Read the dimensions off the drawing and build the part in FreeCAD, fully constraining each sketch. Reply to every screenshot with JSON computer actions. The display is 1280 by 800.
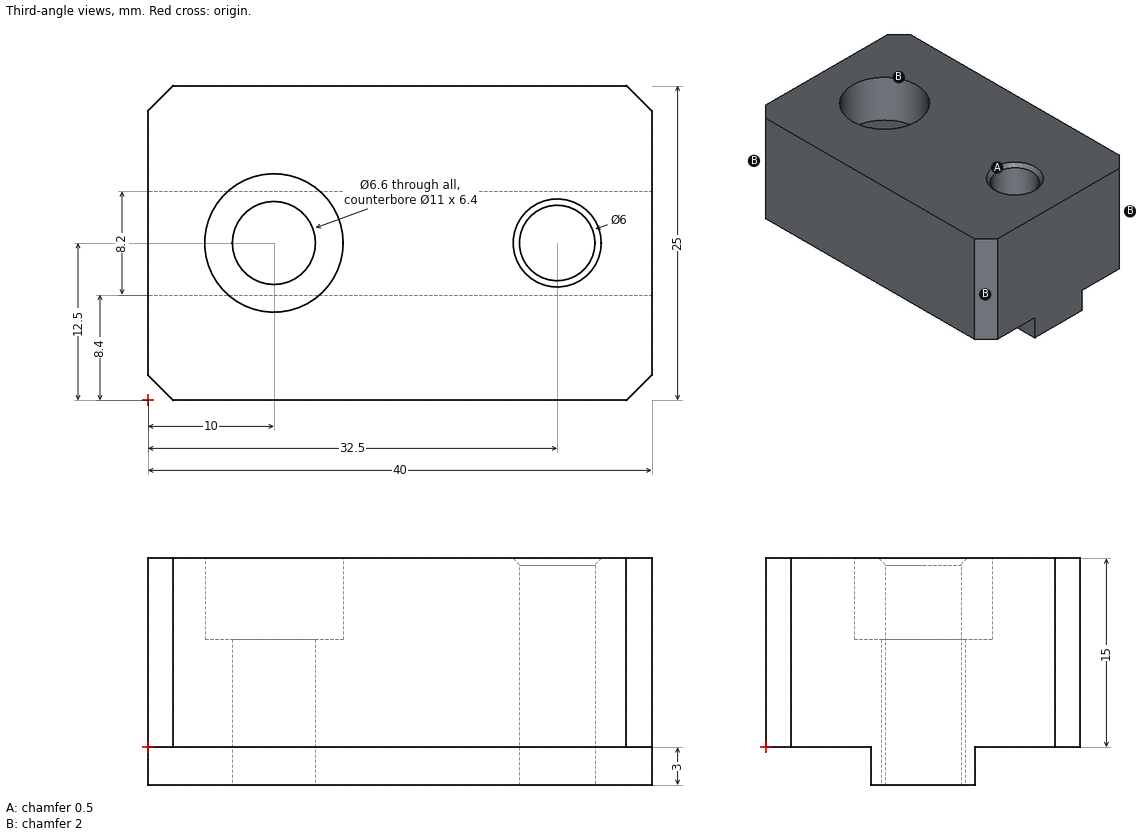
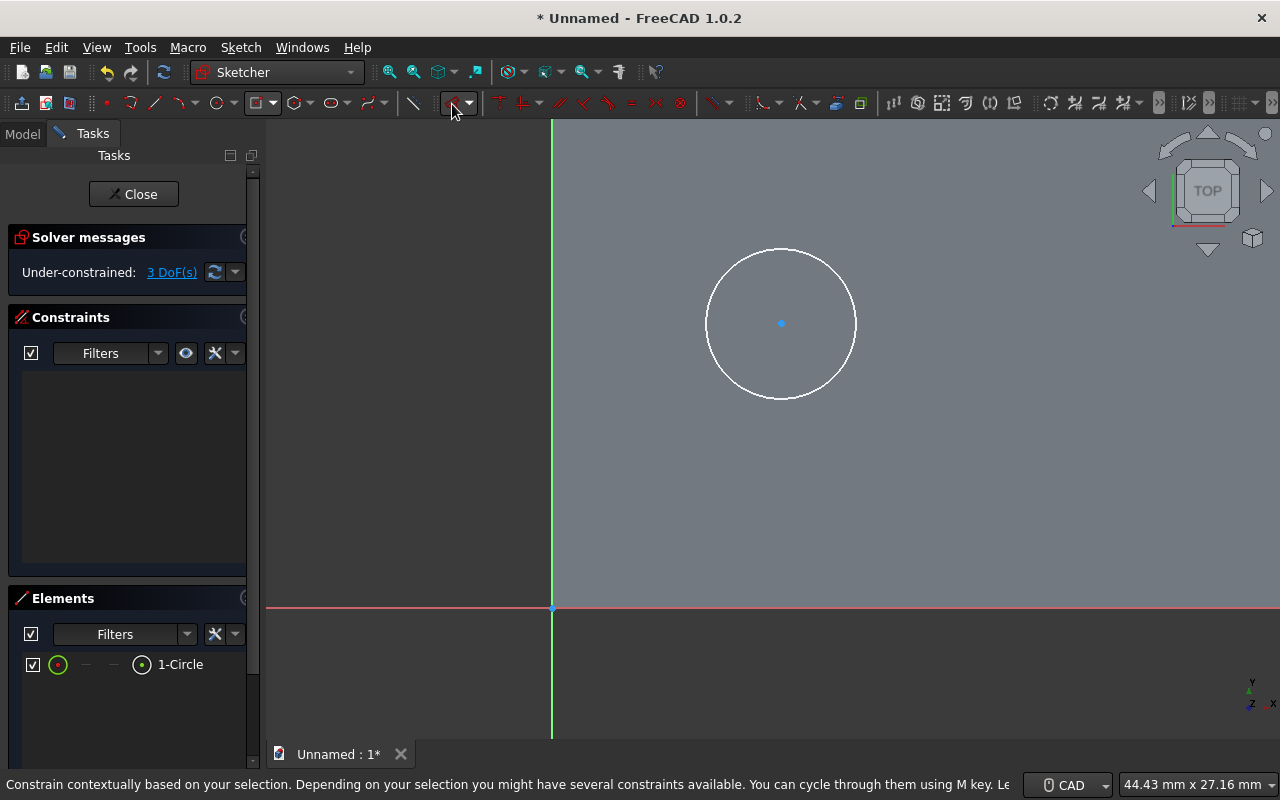
{"action": "left_click", "coordinate": [834, 271]}
{"action": "left_click", "coordinate": [857, 248]}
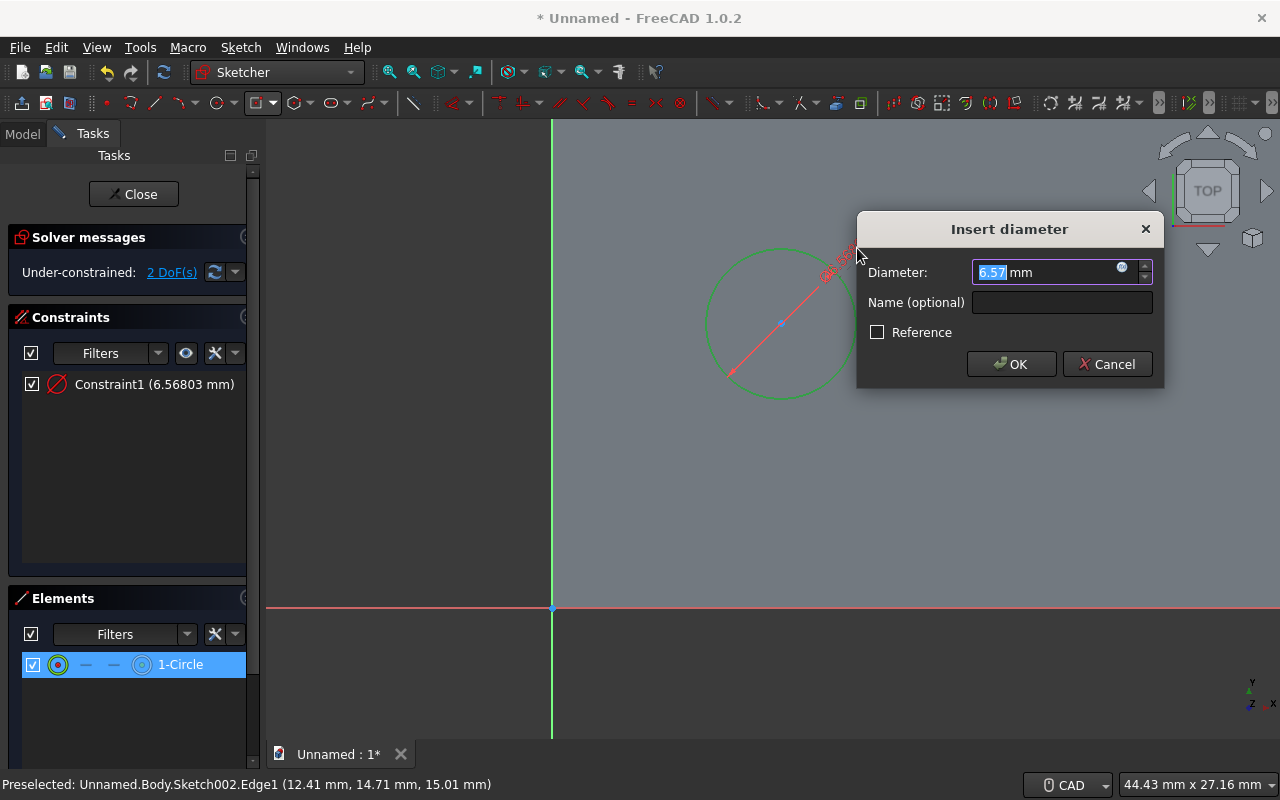
{"action": "type", "text": "6.6"}
{"action": "key", "text": "Return"}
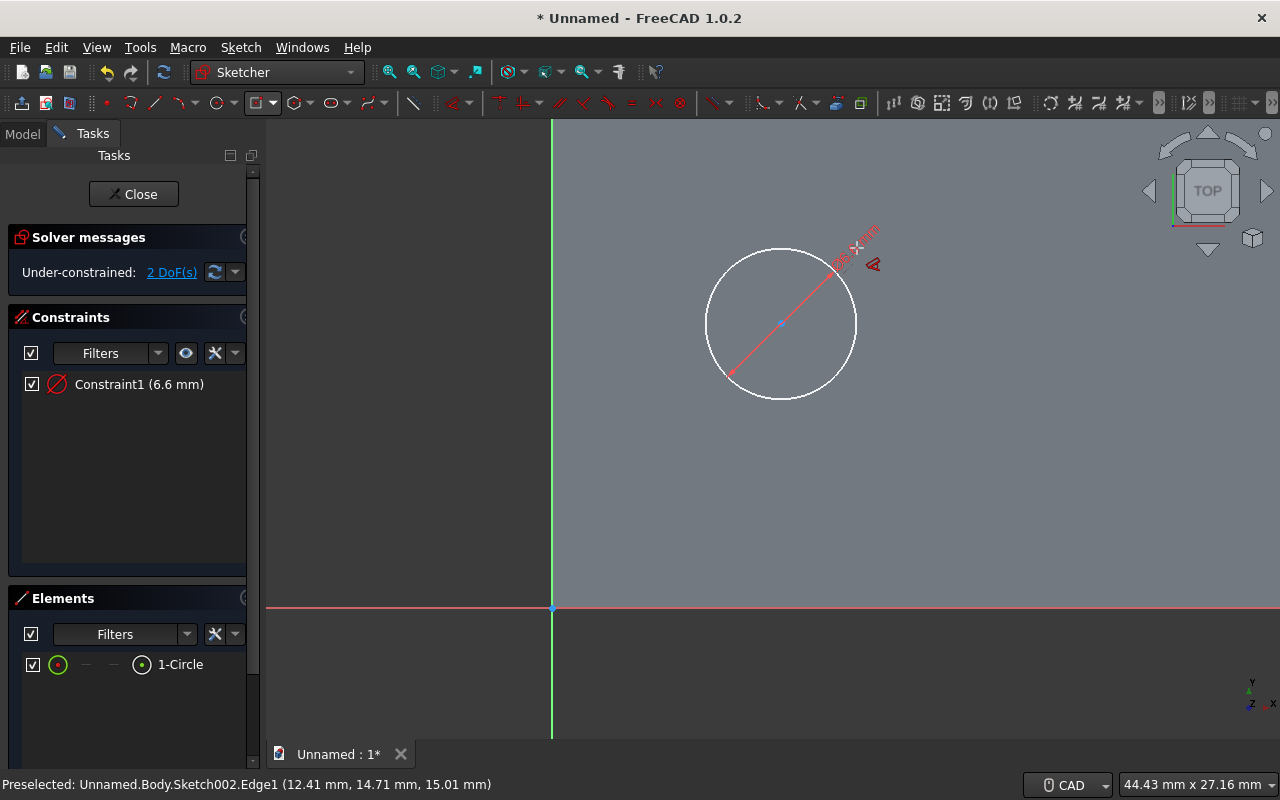
{"action": "left_click", "coordinate": [781, 324]}
{"action": "left_click", "coordinate": [667, 642]}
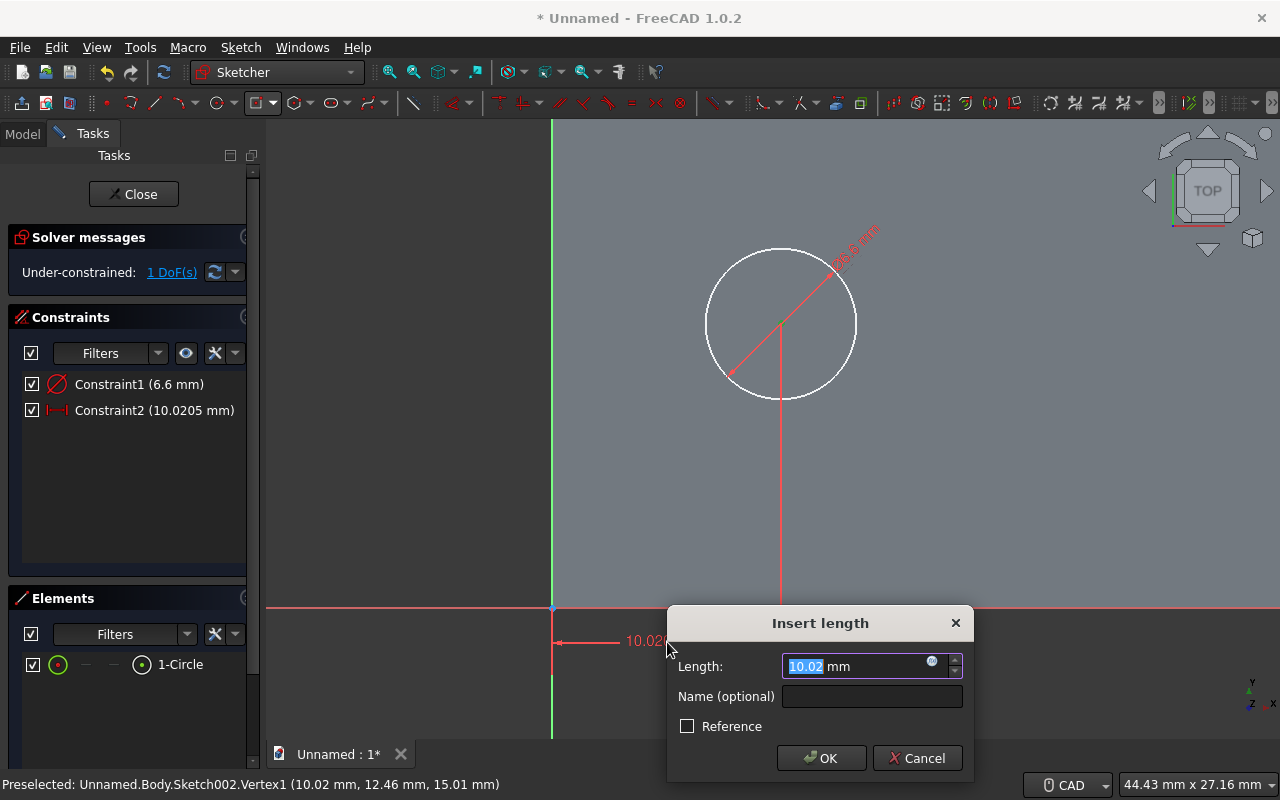
{"action": "type", "text": "10"}
{"action": "key", "text": "Return"}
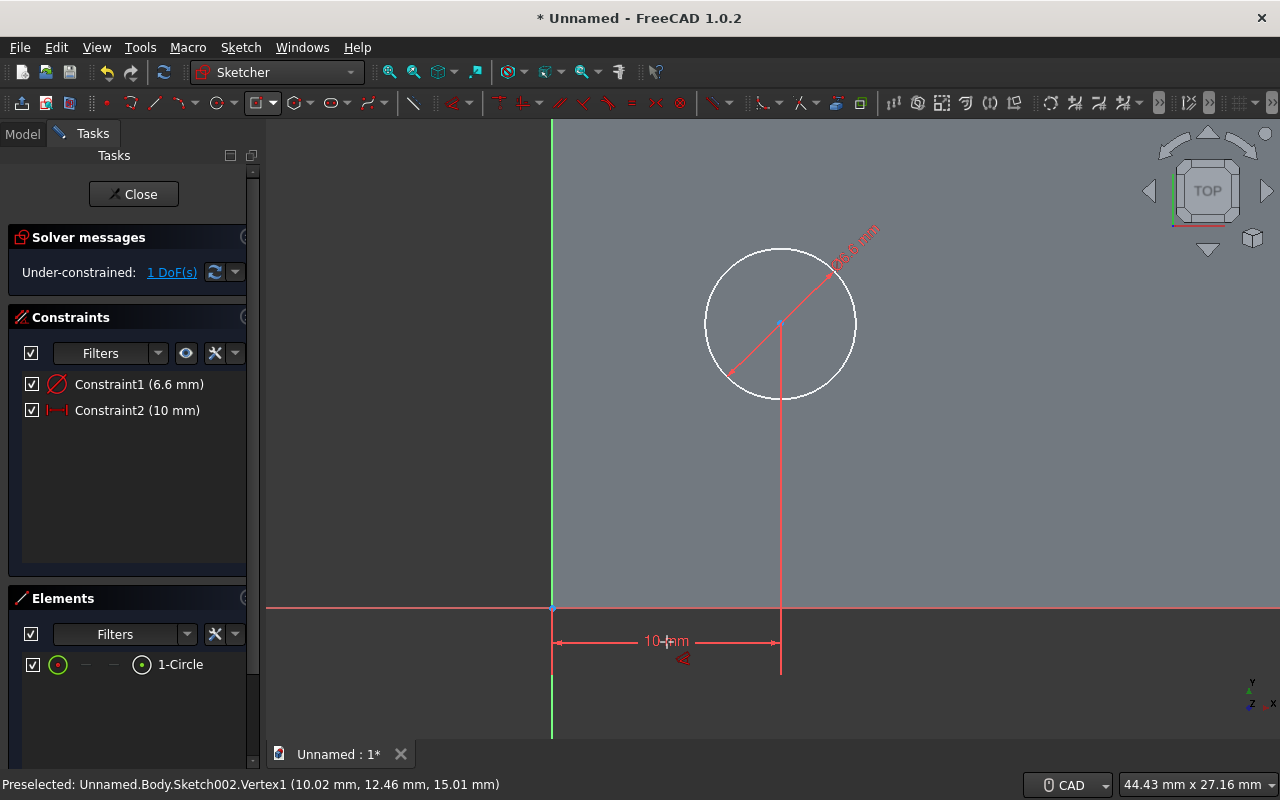
{"action": "left_click", "coordinate": [781, 324]}
{"action": "left_click", "coordinate": [518, 466]}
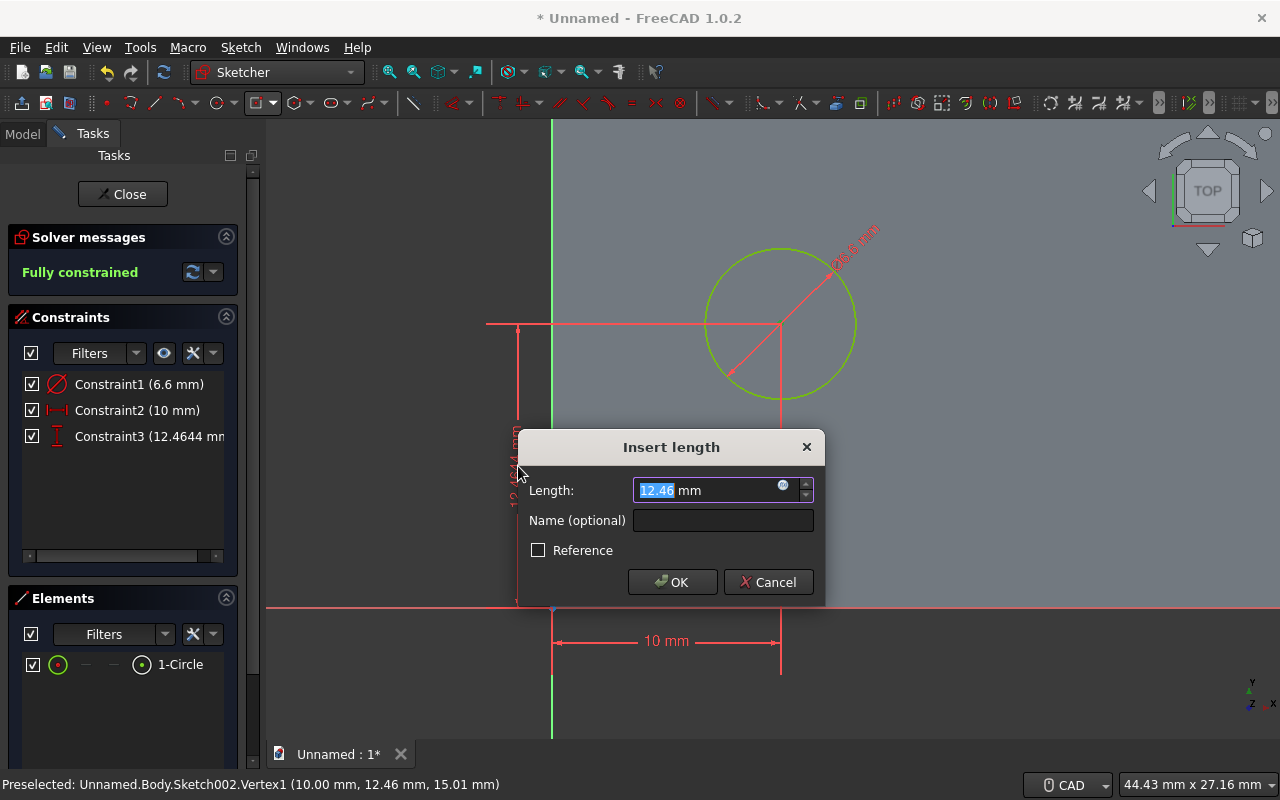
{"action": "type", "text": "12.5"}
{"action": "key", "text": "Return"}
{"action": "key", "text": "Escape"}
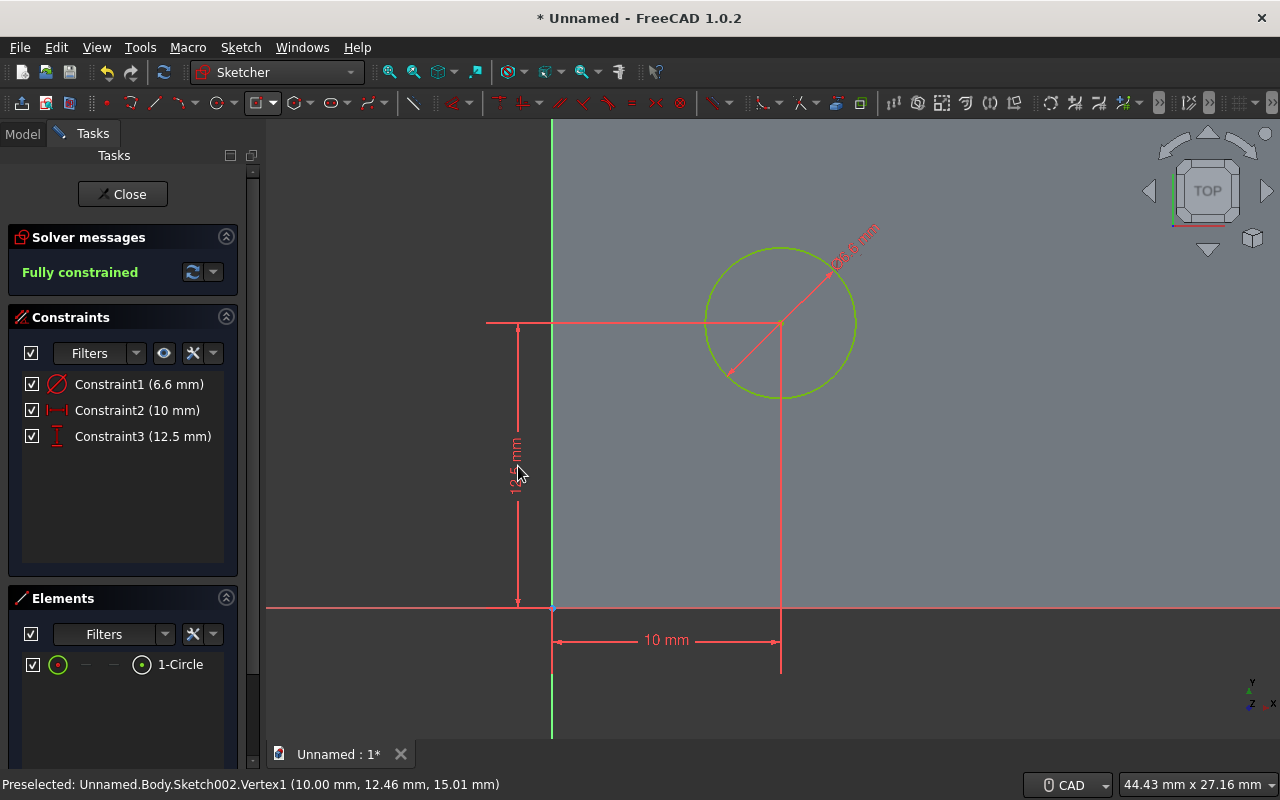
{"action": "left_click", "coordinate": [123, 194]}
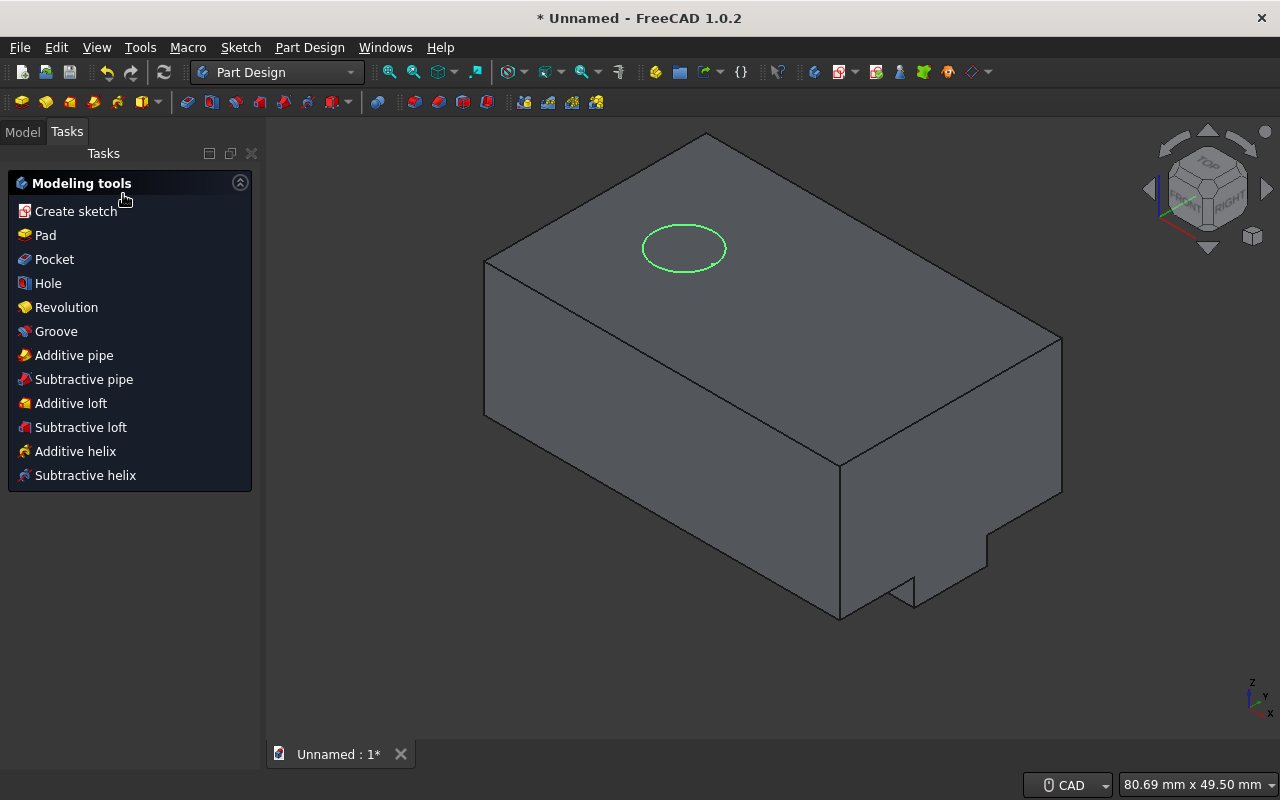
{"action": "left_click", "coordinate": [212, 102]}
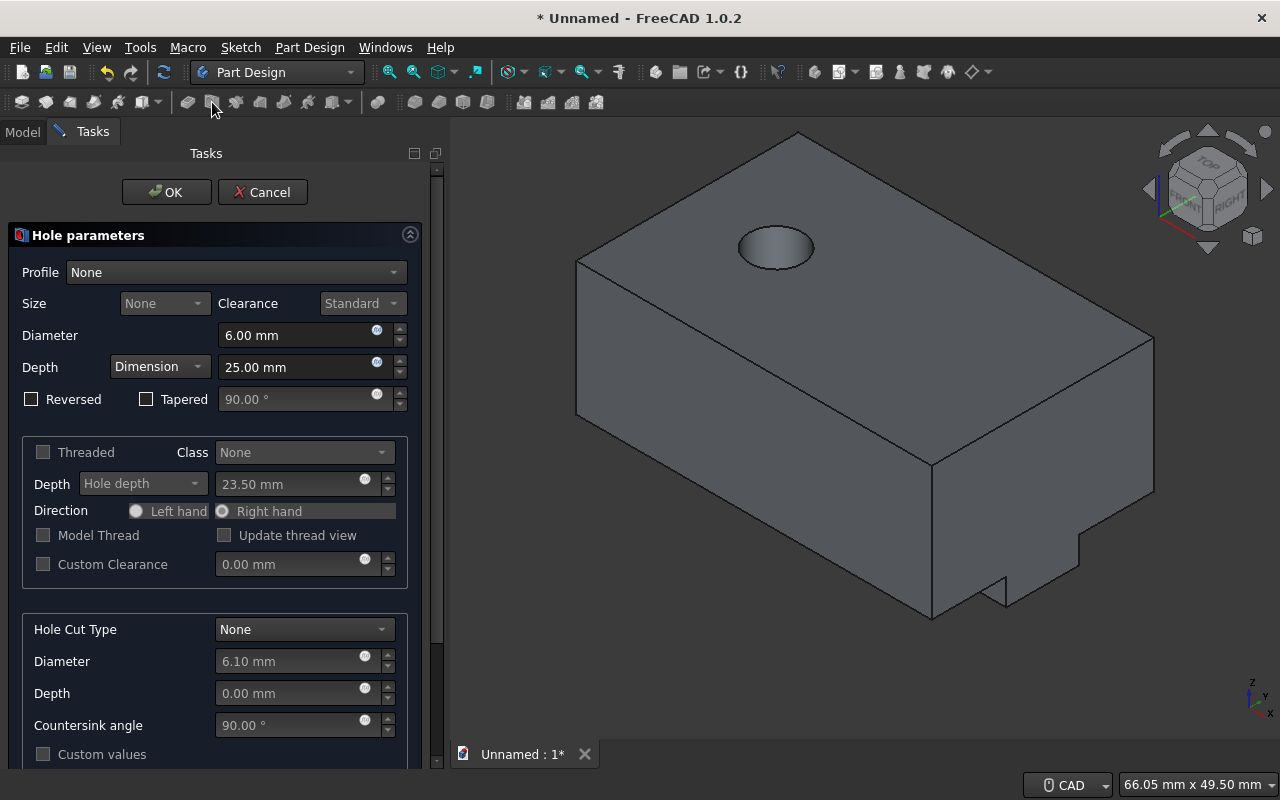
{"action": "triple_click", "coordinate": [305, 335]}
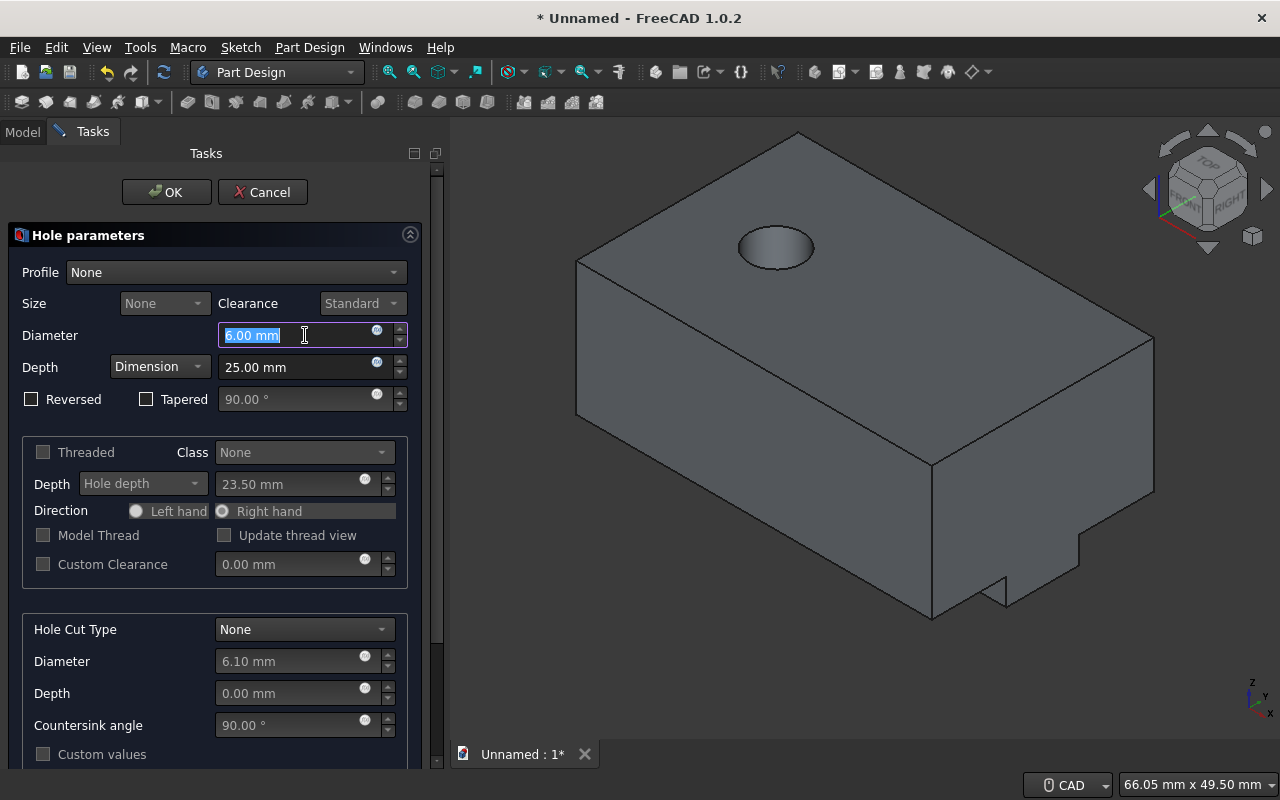
{"action": "type", "text": "6.6"}
{"action": "key", "text": "Tab"}